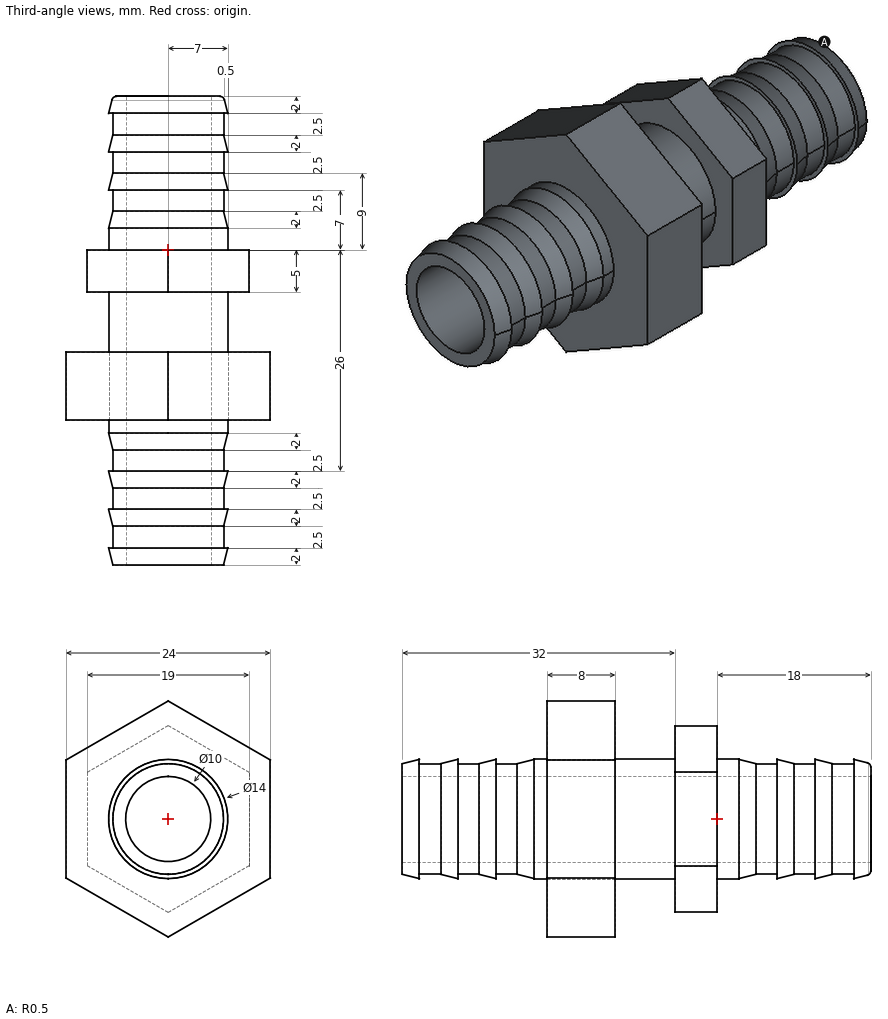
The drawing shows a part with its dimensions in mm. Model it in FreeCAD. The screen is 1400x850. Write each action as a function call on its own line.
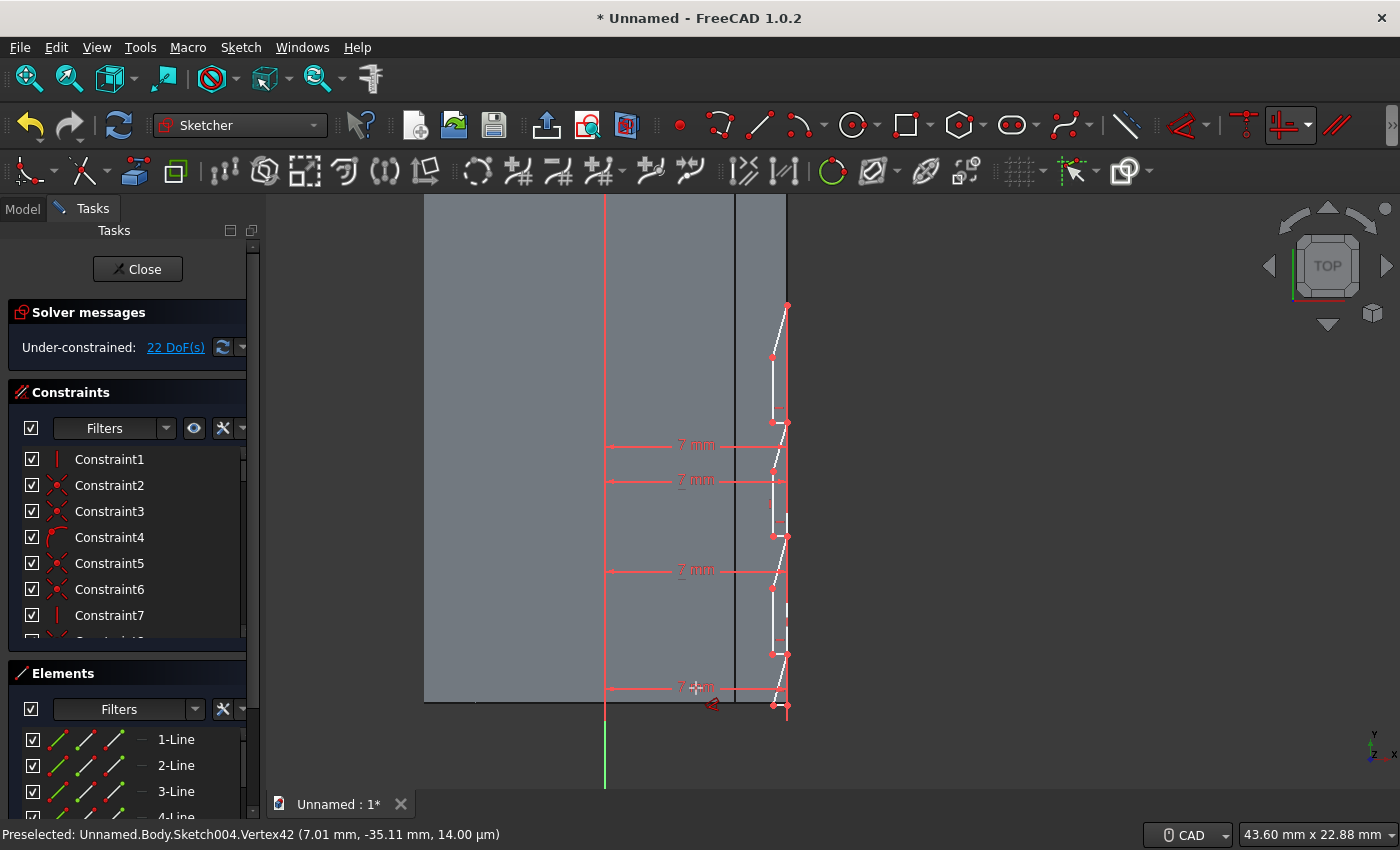
scroll(787, 656, down, 7)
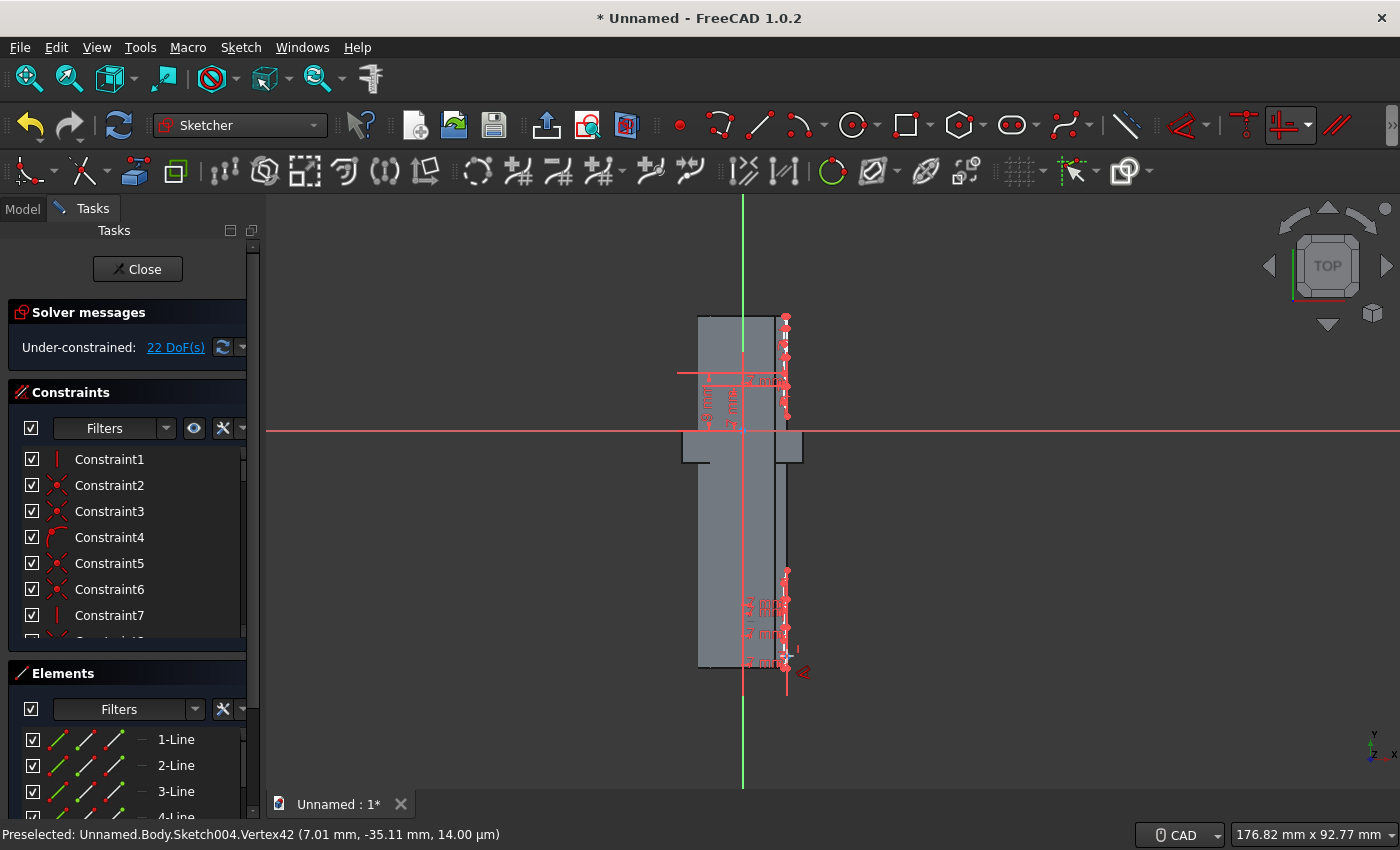
scroll(785, 320, up, 10)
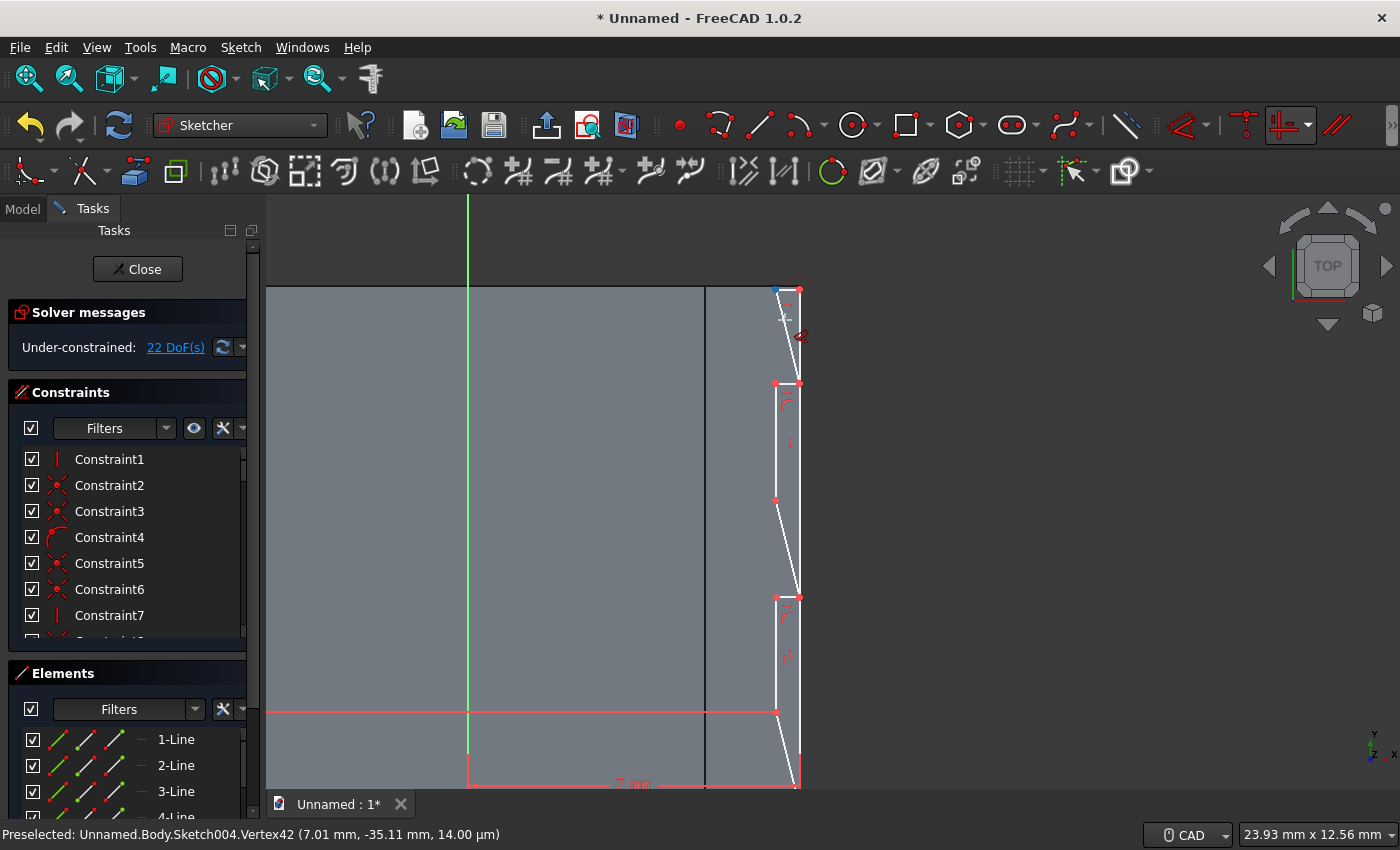
click(783, 318)
click(834, 337)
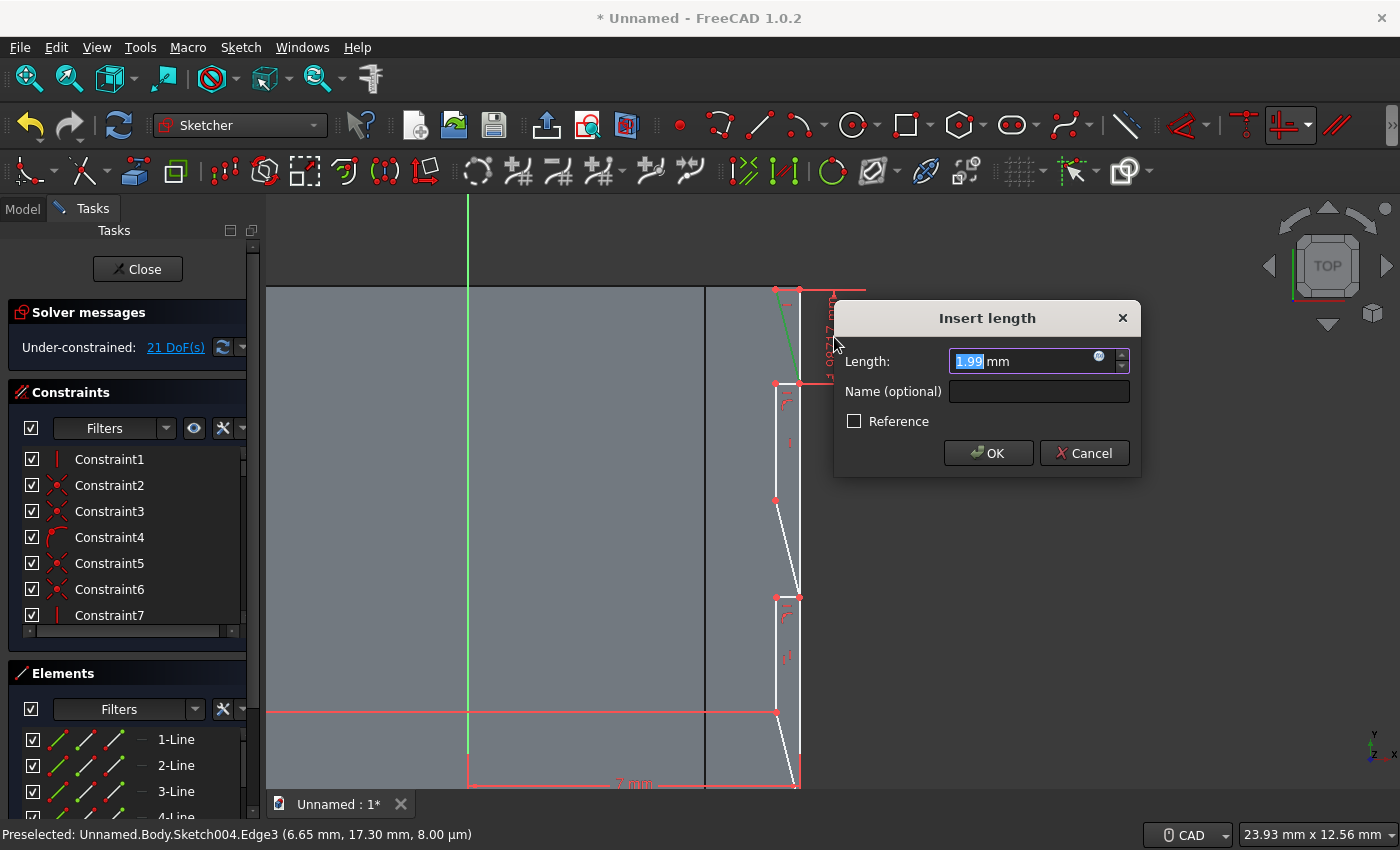
text(2)
key(Return)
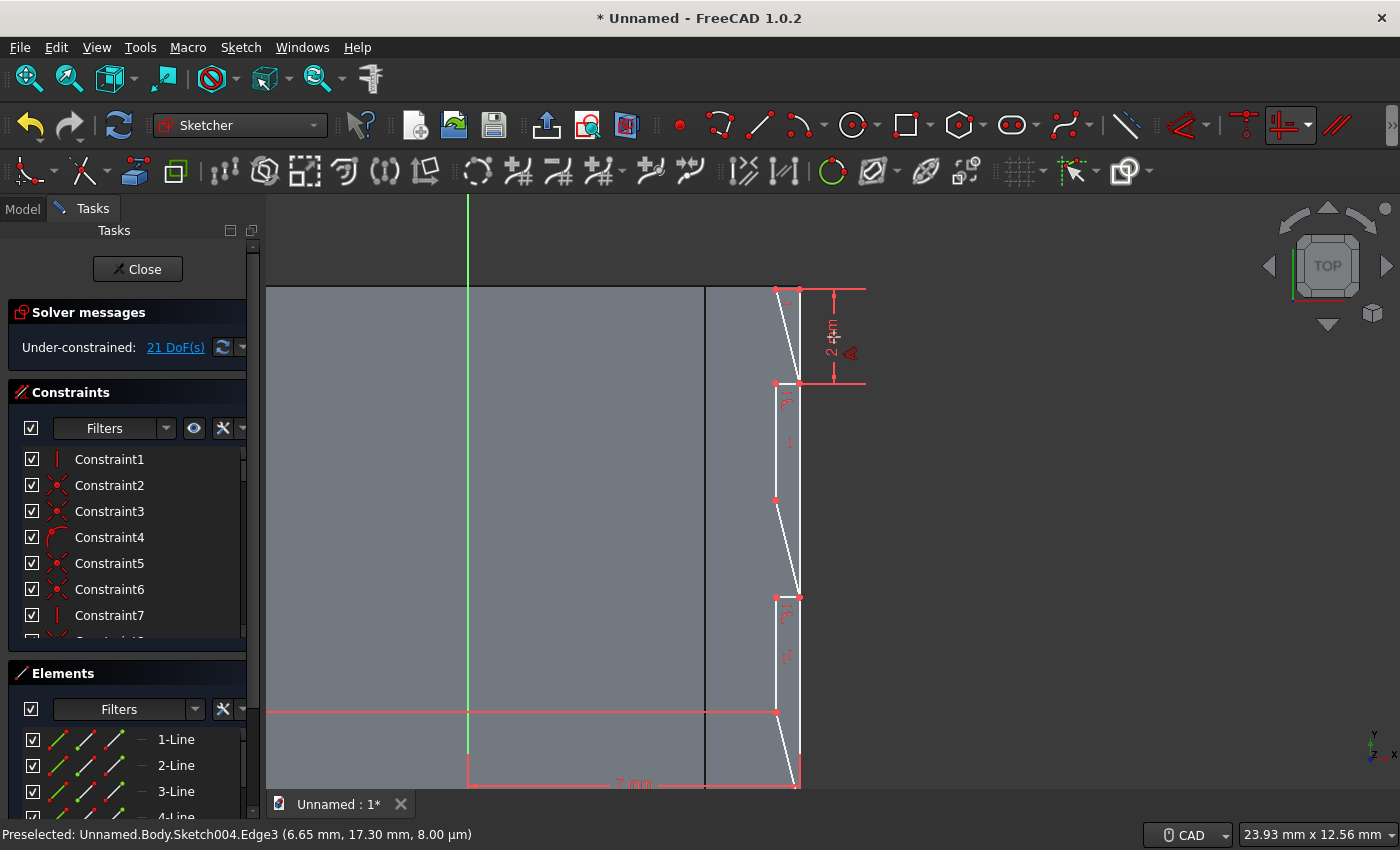
click(783, 530)
click(834, 549)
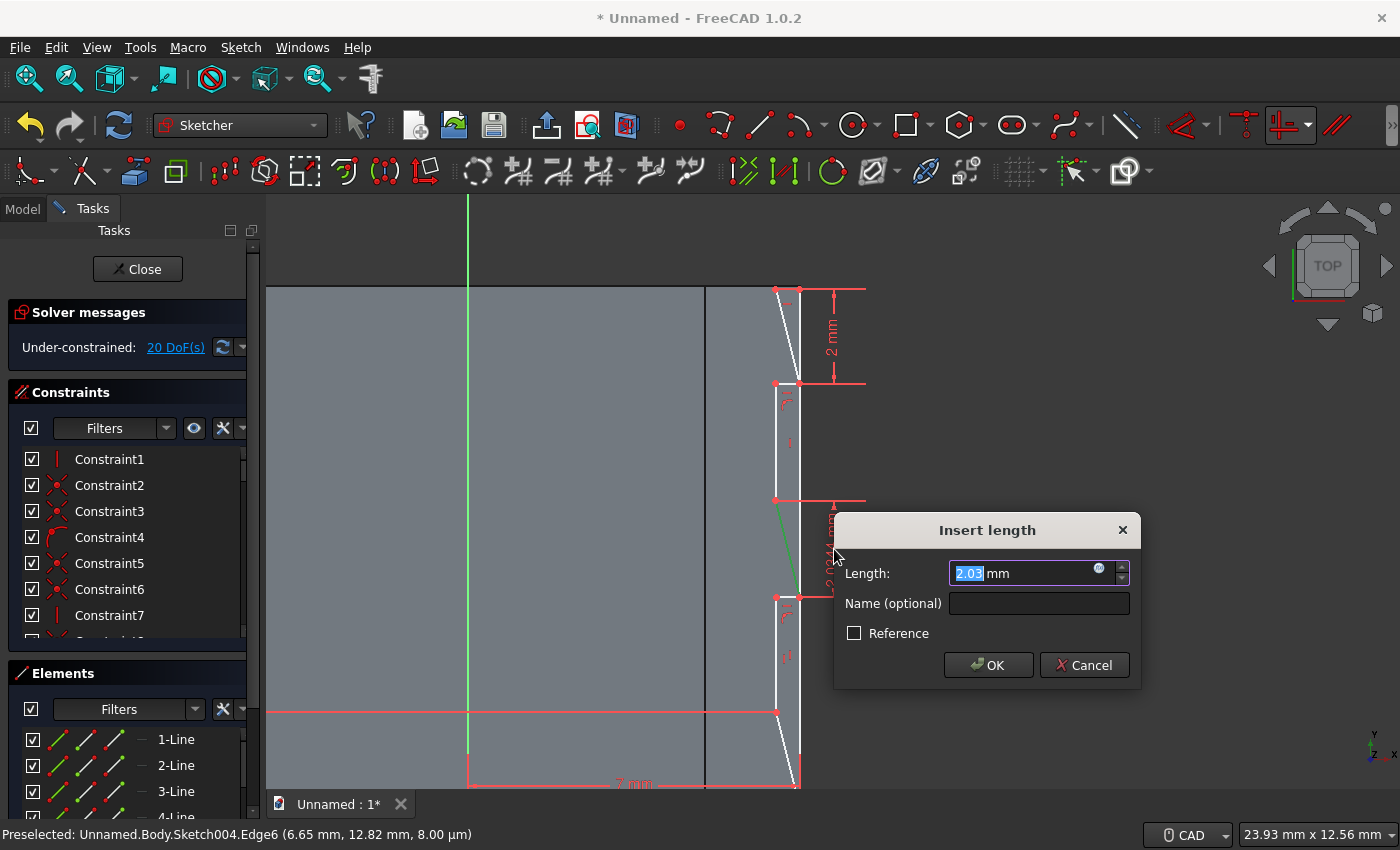
text(2)
key(Return)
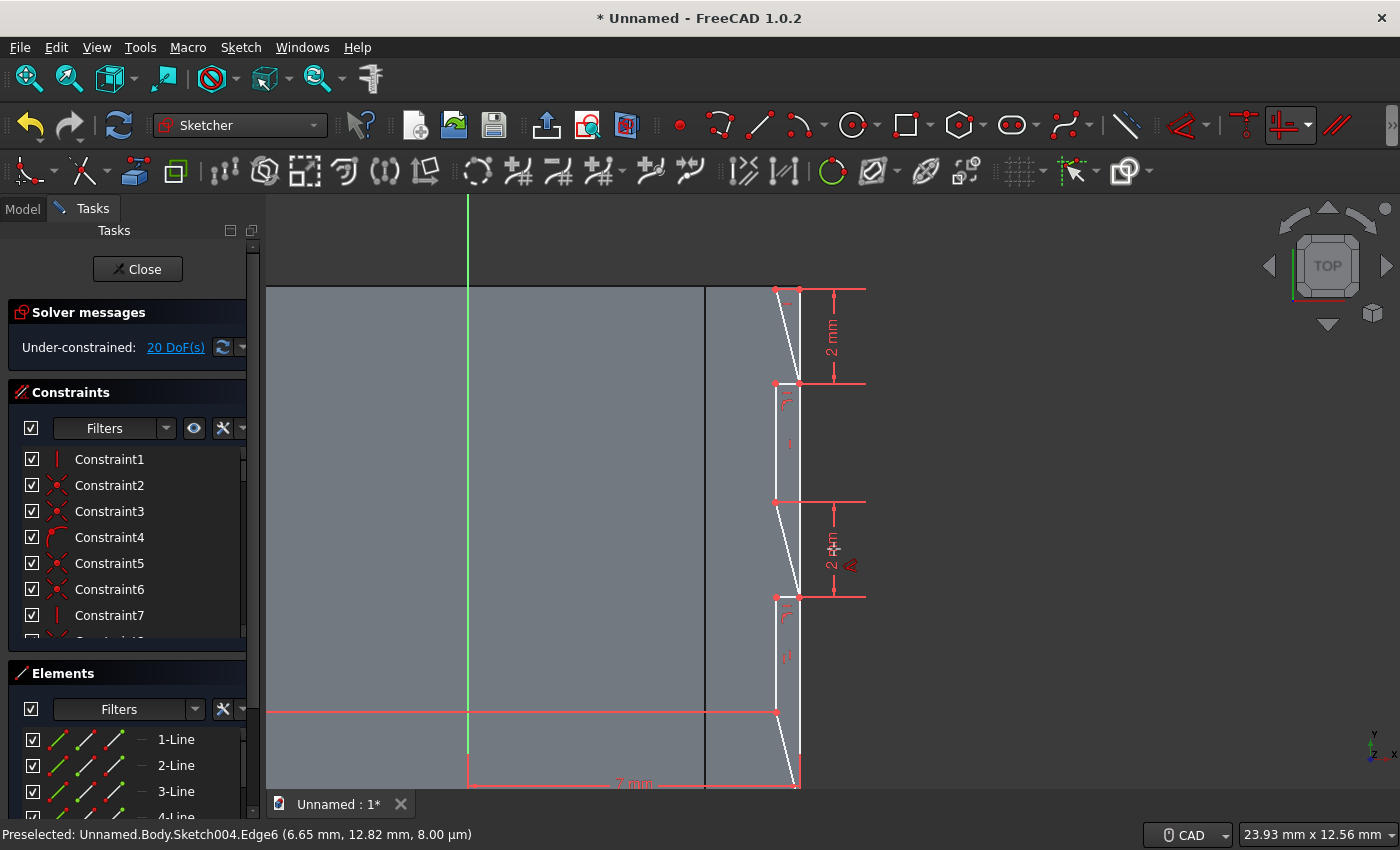
scroll(785, 320, down, 10)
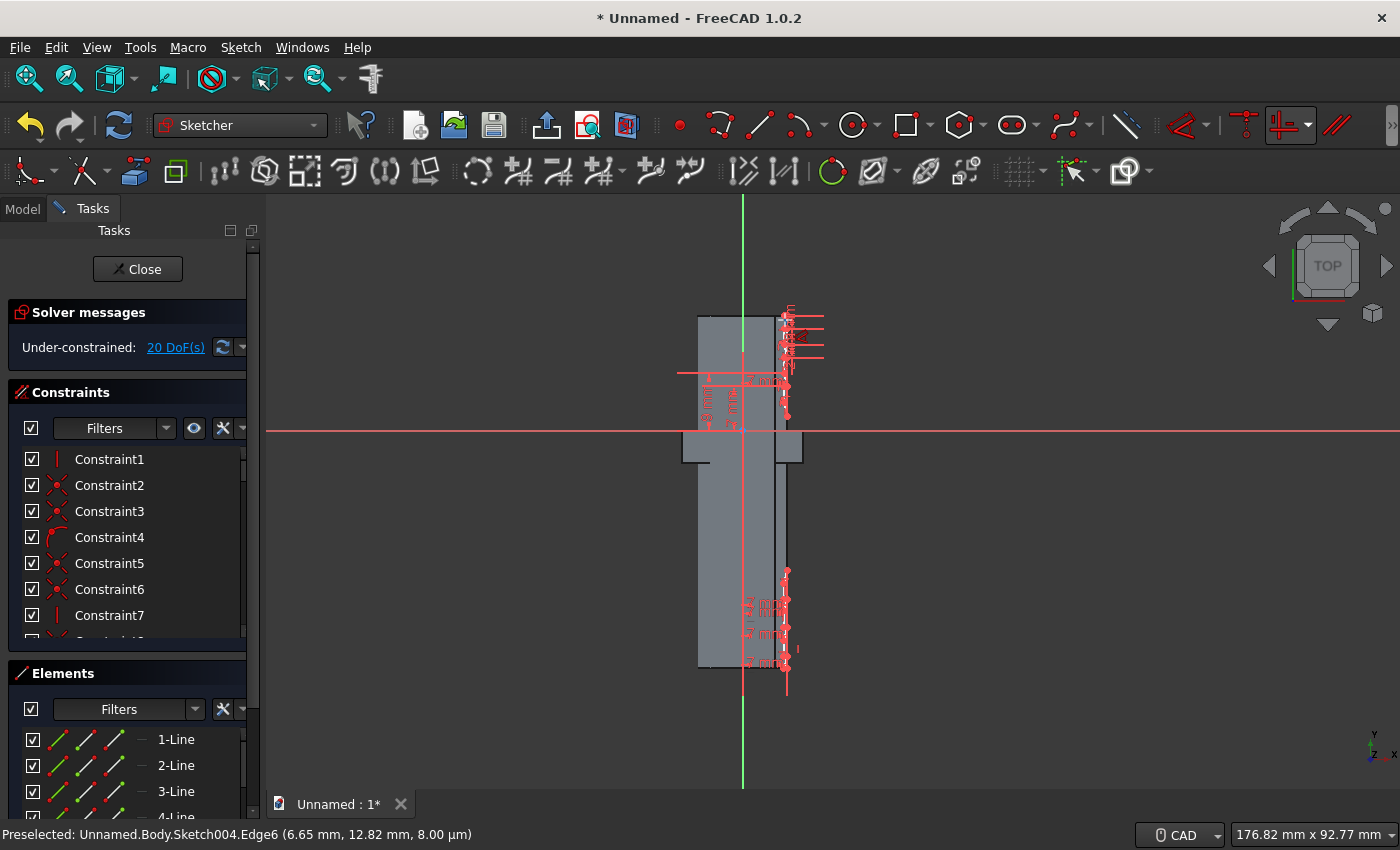
scroll(785, 406, up, 10)